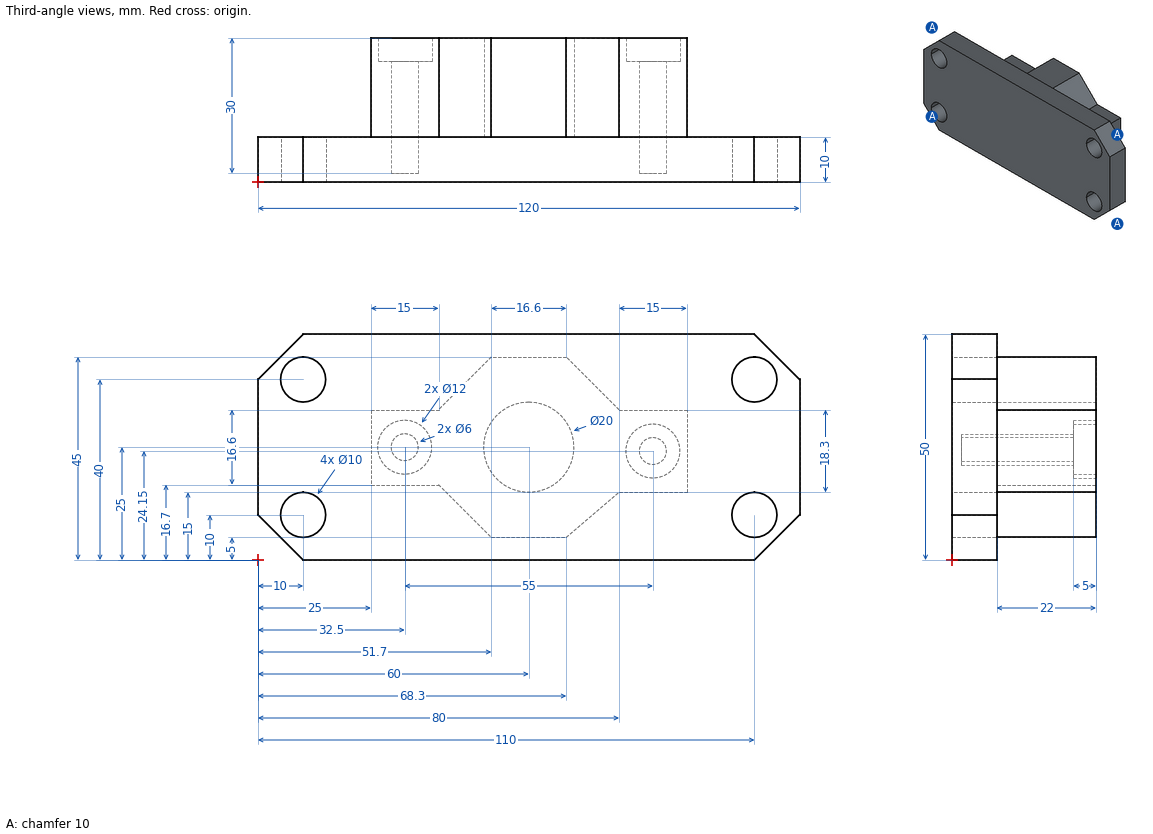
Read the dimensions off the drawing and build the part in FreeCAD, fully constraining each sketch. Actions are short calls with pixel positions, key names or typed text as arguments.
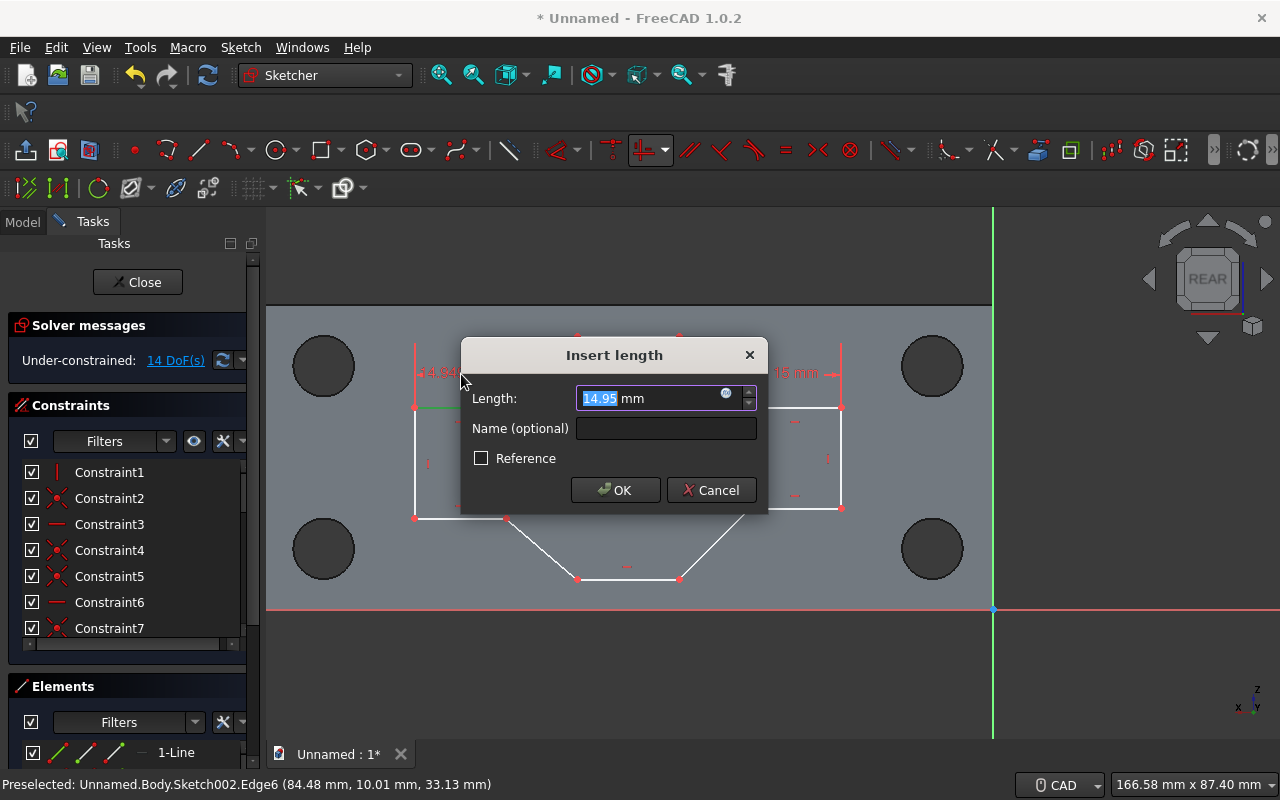
text(15)
key(Return)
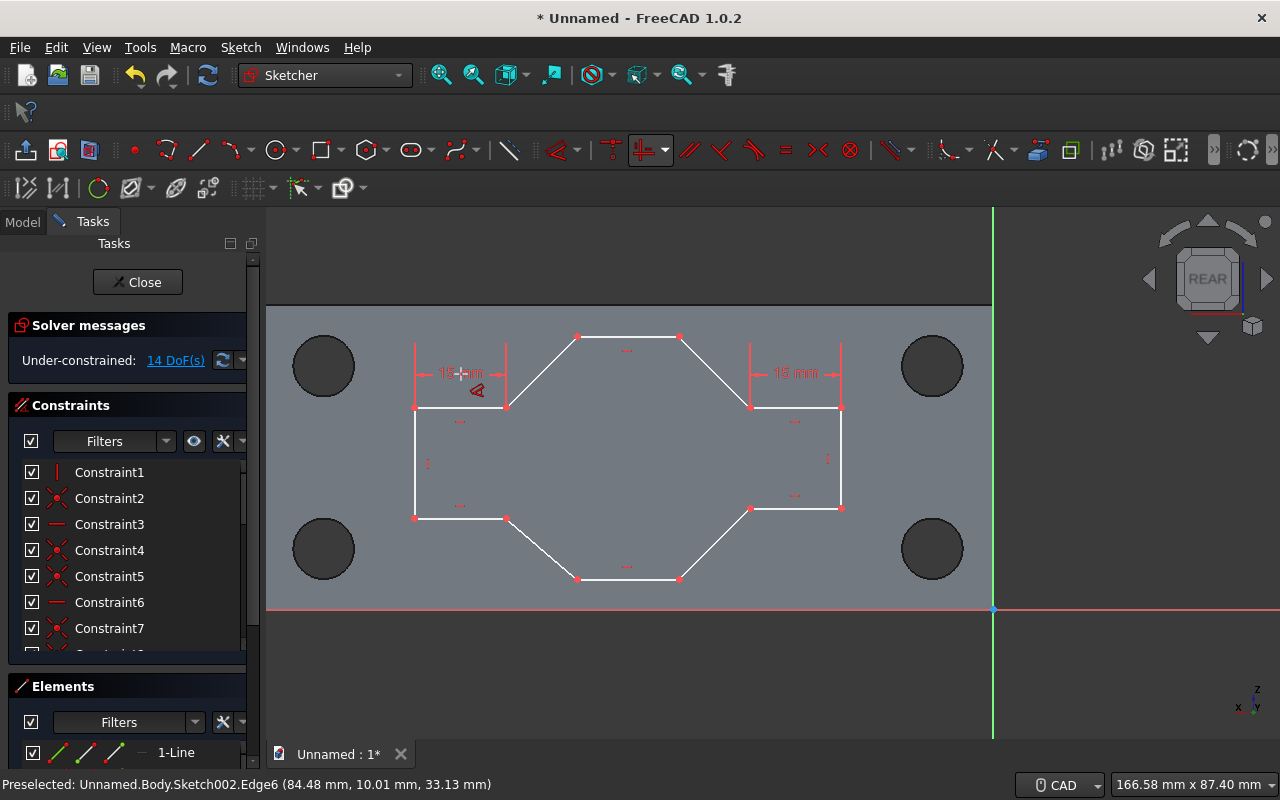
click(442, 519)
click(461, 553)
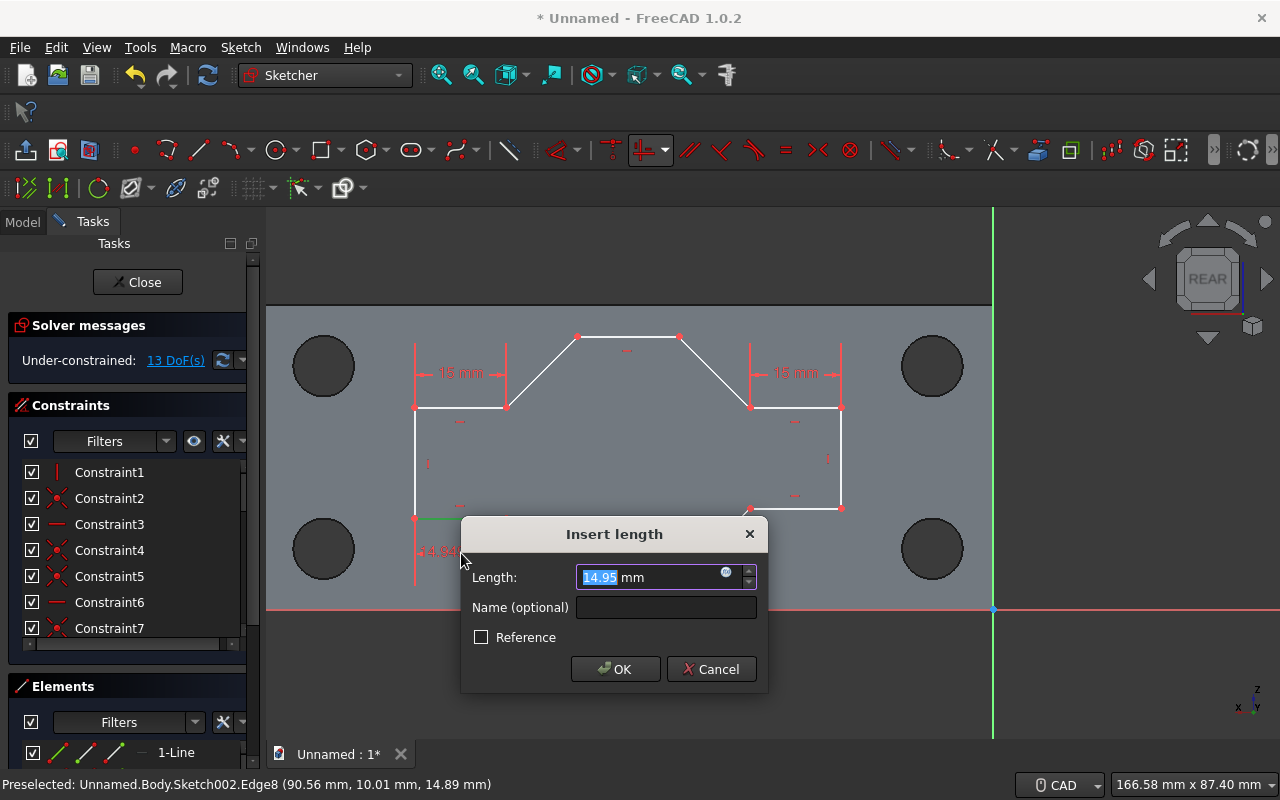
text(15)
key(Return)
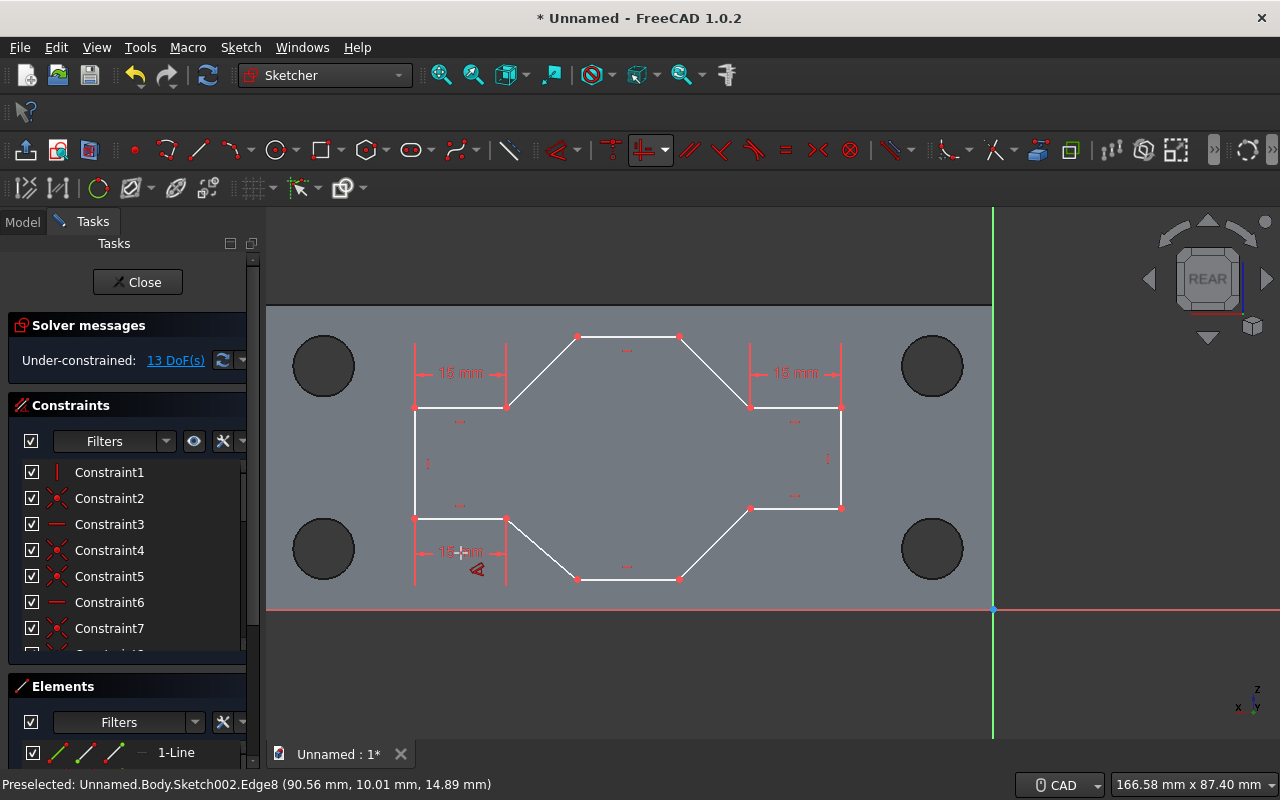
click(777, 509)
click(796, 543)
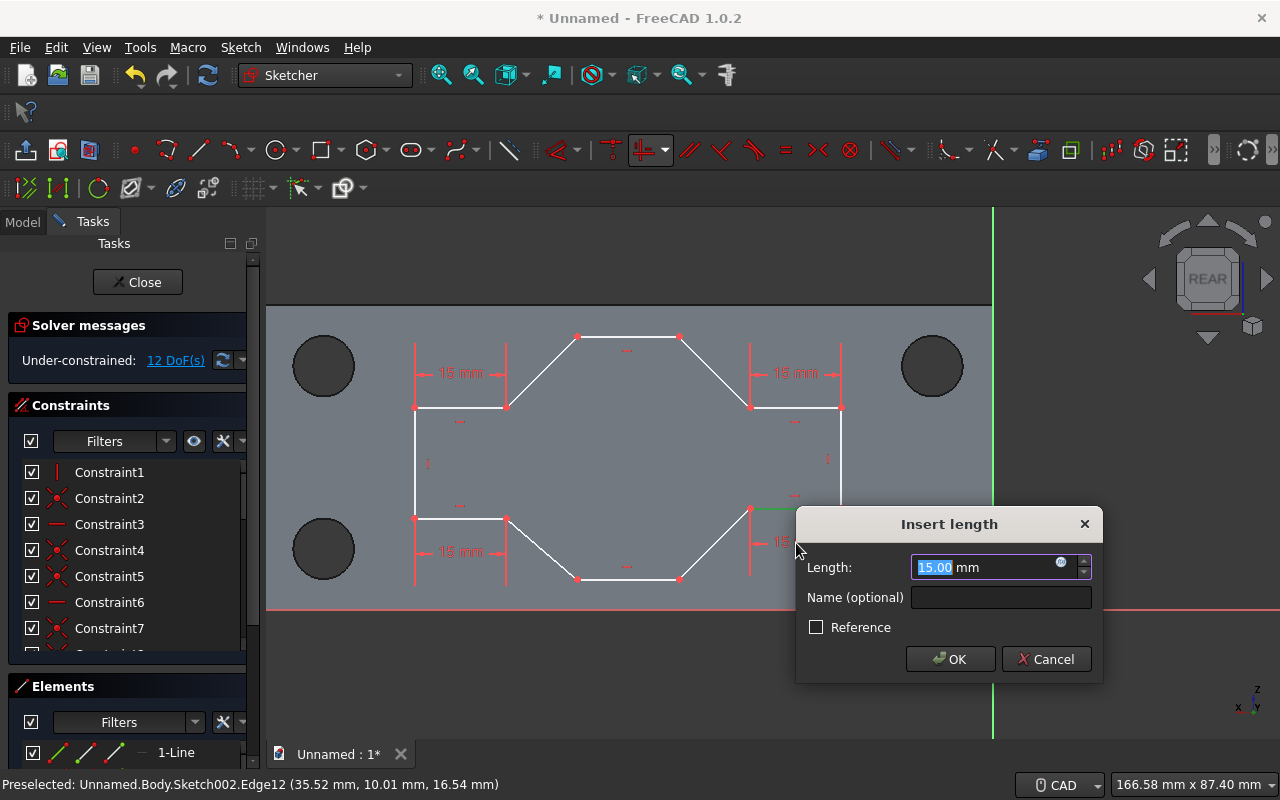
text(15)
key(Return)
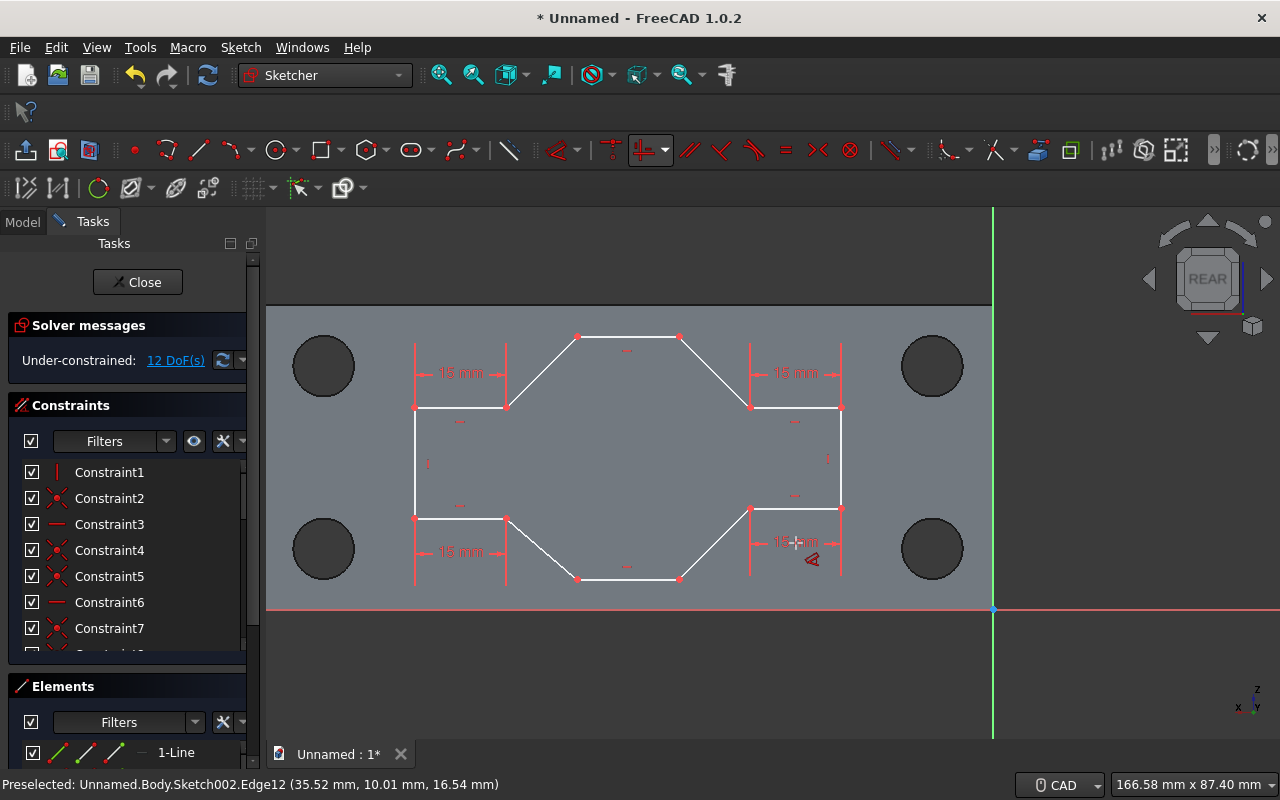
scroll(577, 580, up, 2)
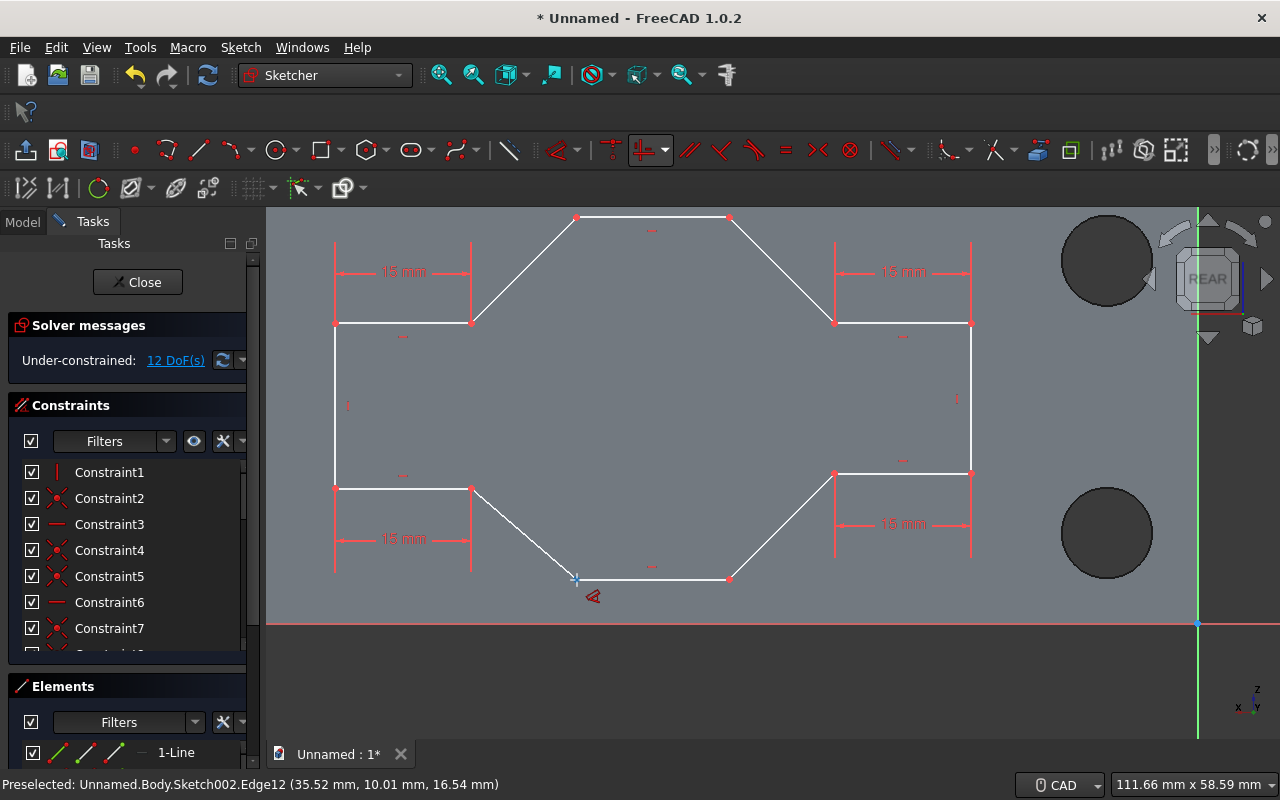
click(577, 580)
click(543, 602)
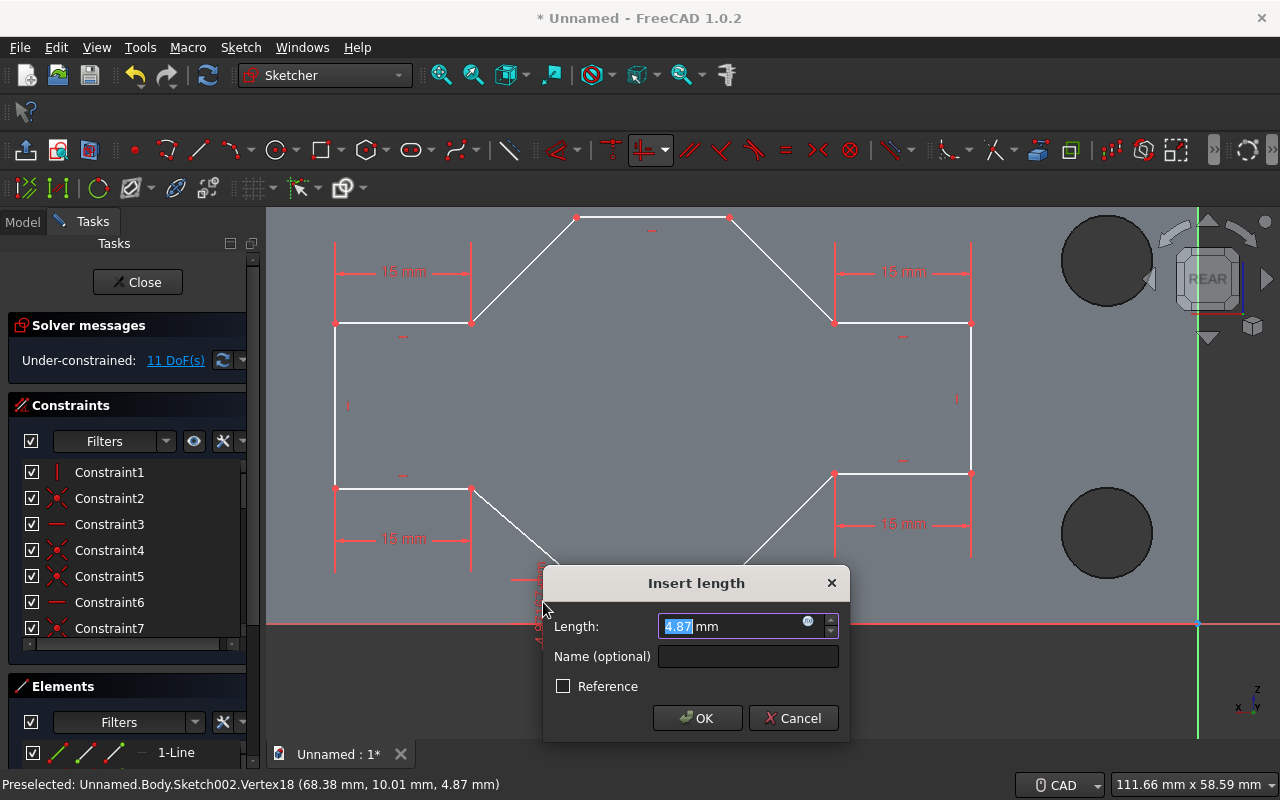
text(5)
key(Return)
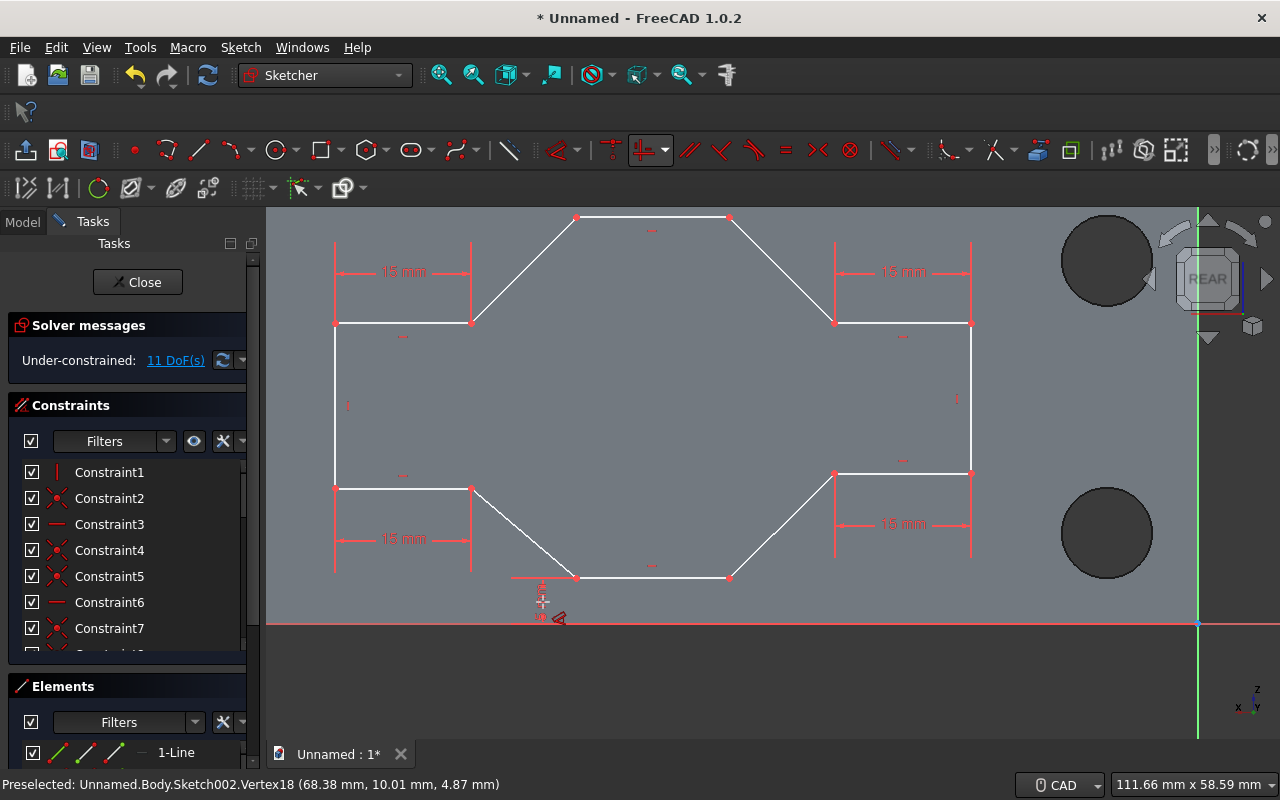
click(971, 474)
click(1043, 658)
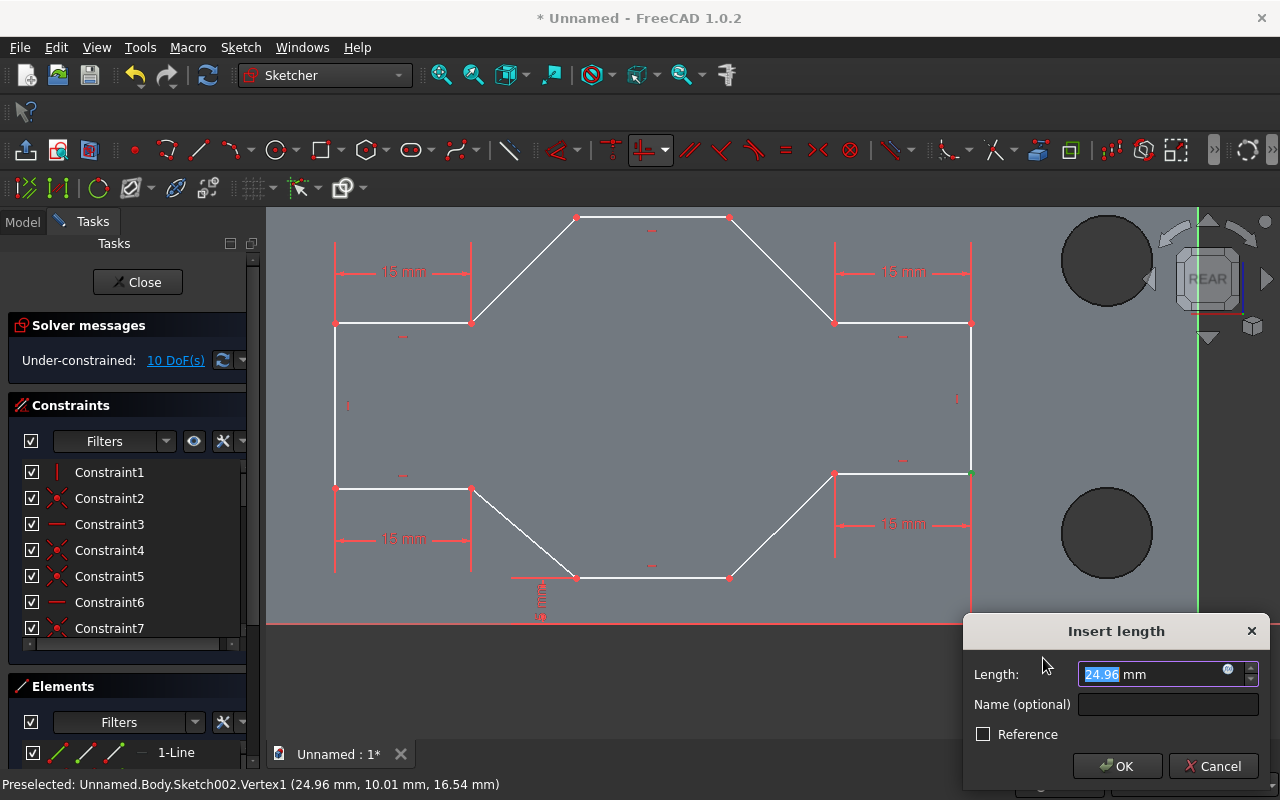
text(25)
key(Return)